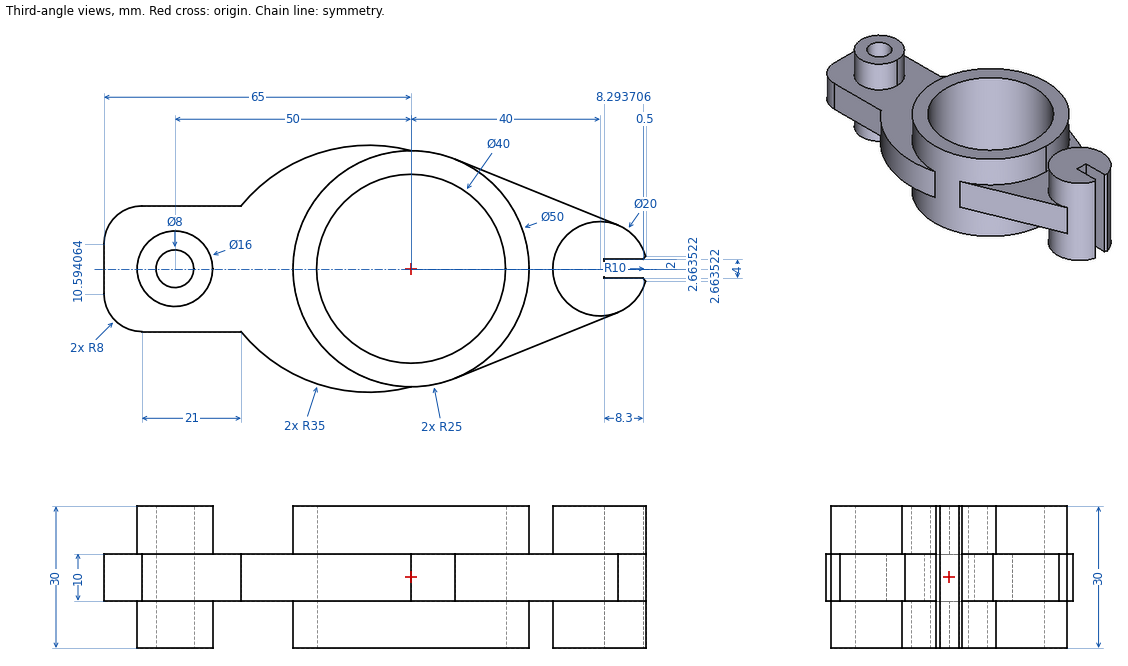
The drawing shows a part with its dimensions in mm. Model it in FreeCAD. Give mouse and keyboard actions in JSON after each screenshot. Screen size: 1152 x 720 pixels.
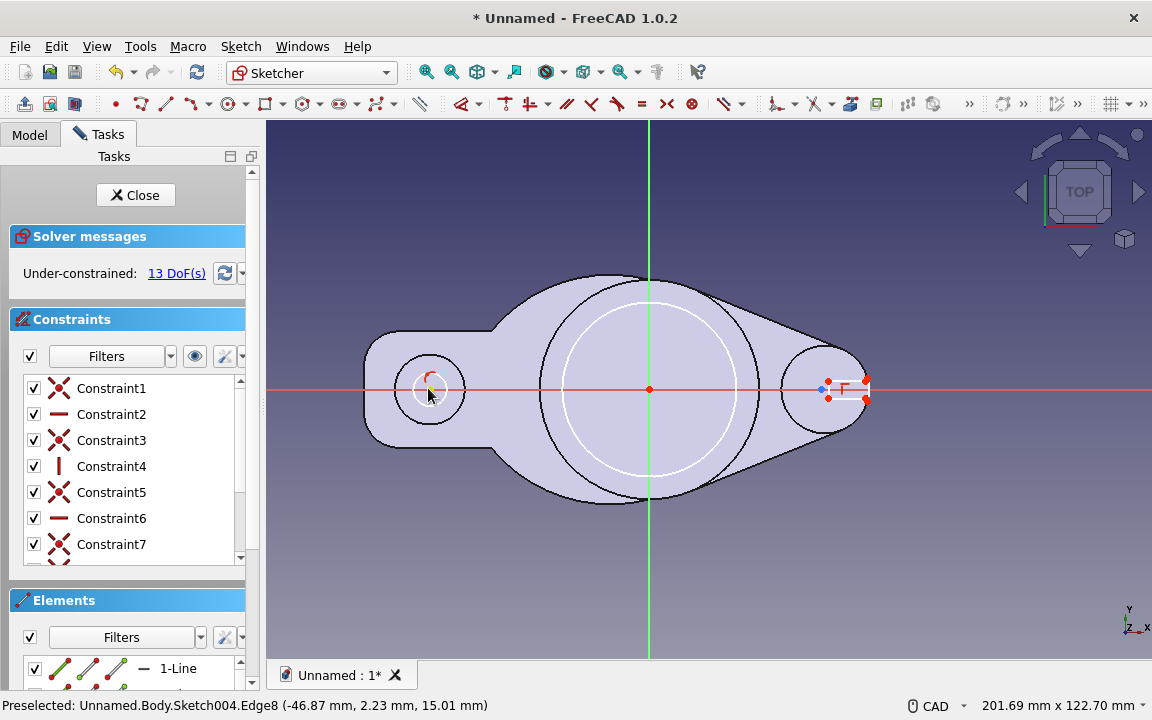
{"action": "left_click", "coordinate": [822, 389]}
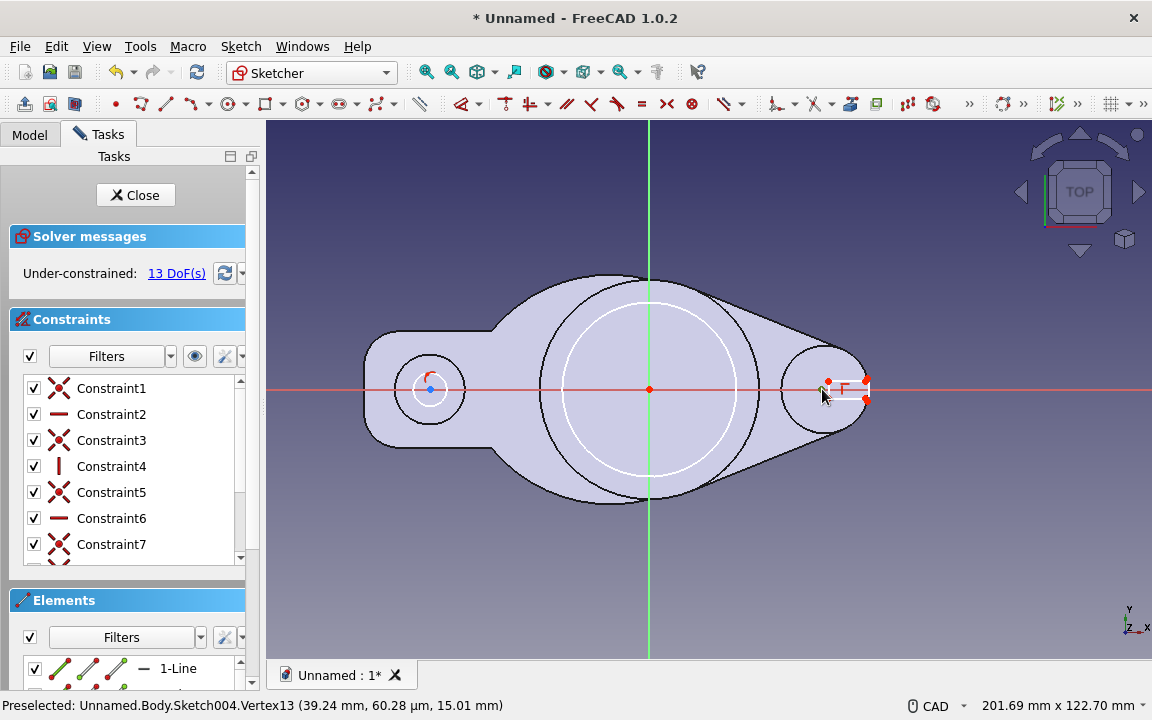
{"action": "left_click", "coordinate": [344, 390]}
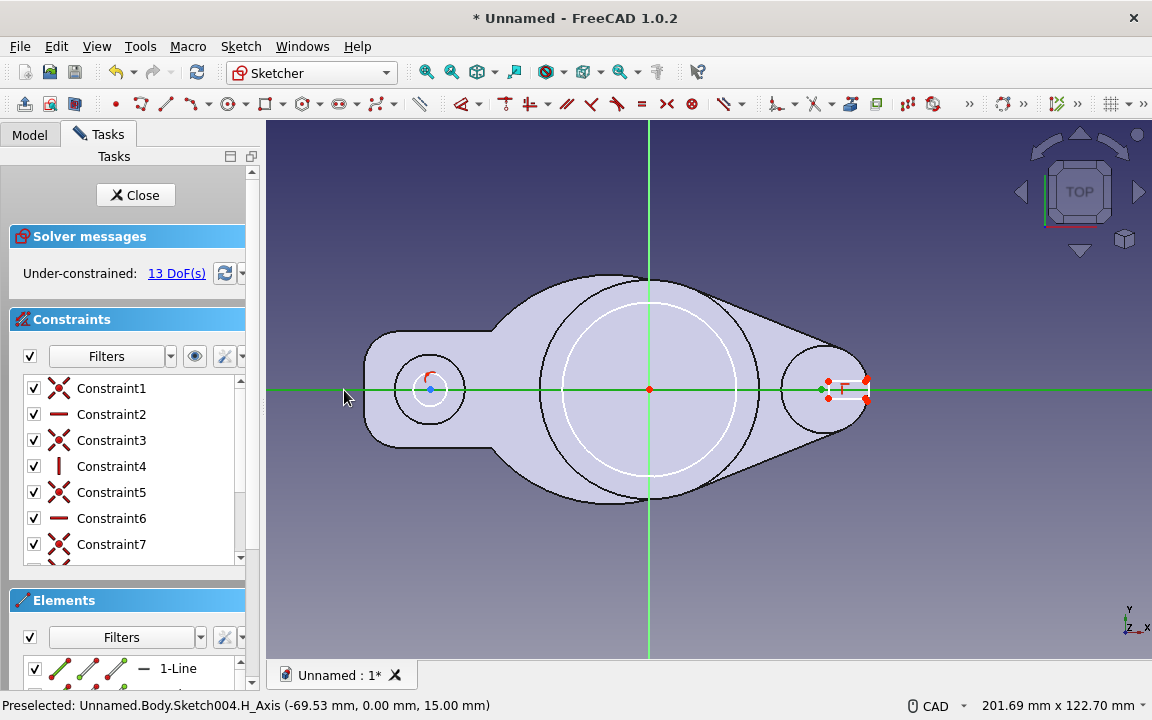
{"action": "left_click", "coordinate": [505, 104]}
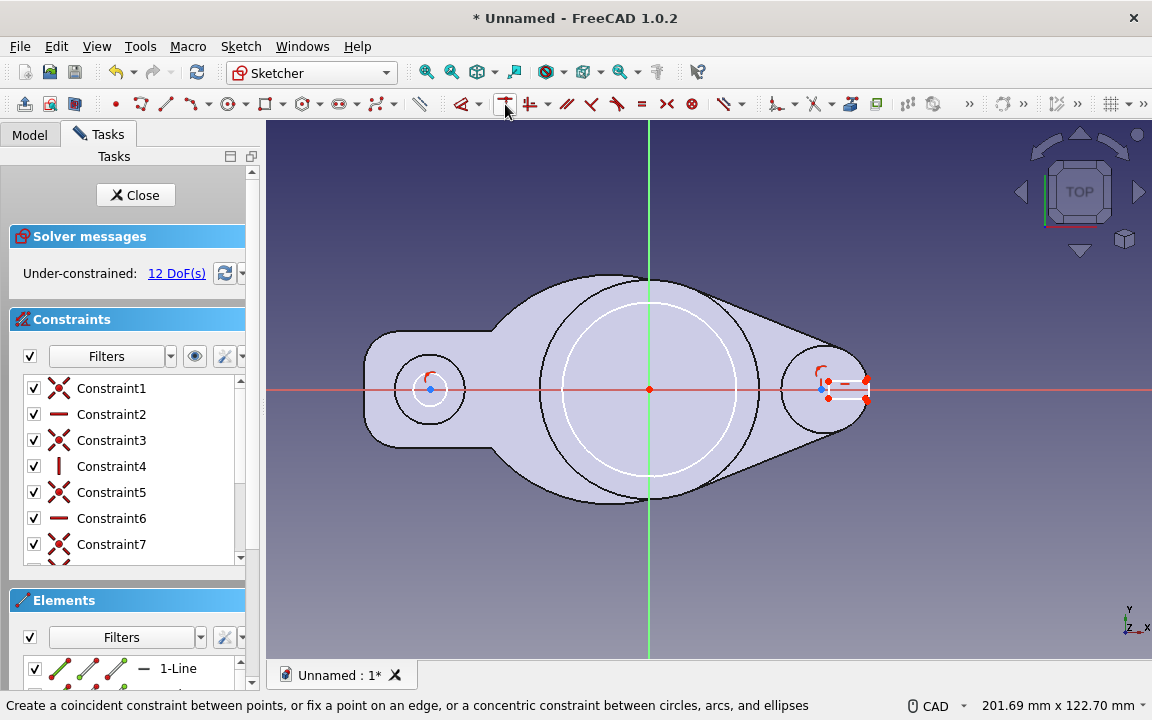
{"action": "left_click", "coordinate": [460, 104]}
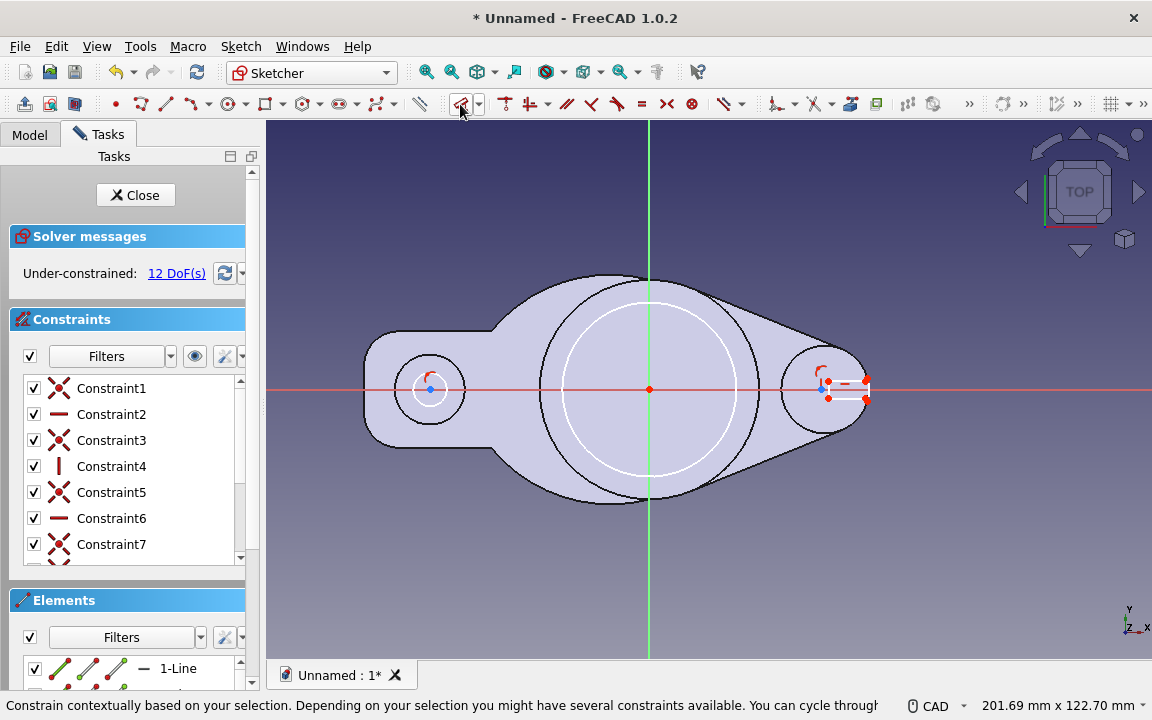
{"action": "scroll", "coordinate": [869, 390], "scroll_direction": "up", "scroll_amount": 2}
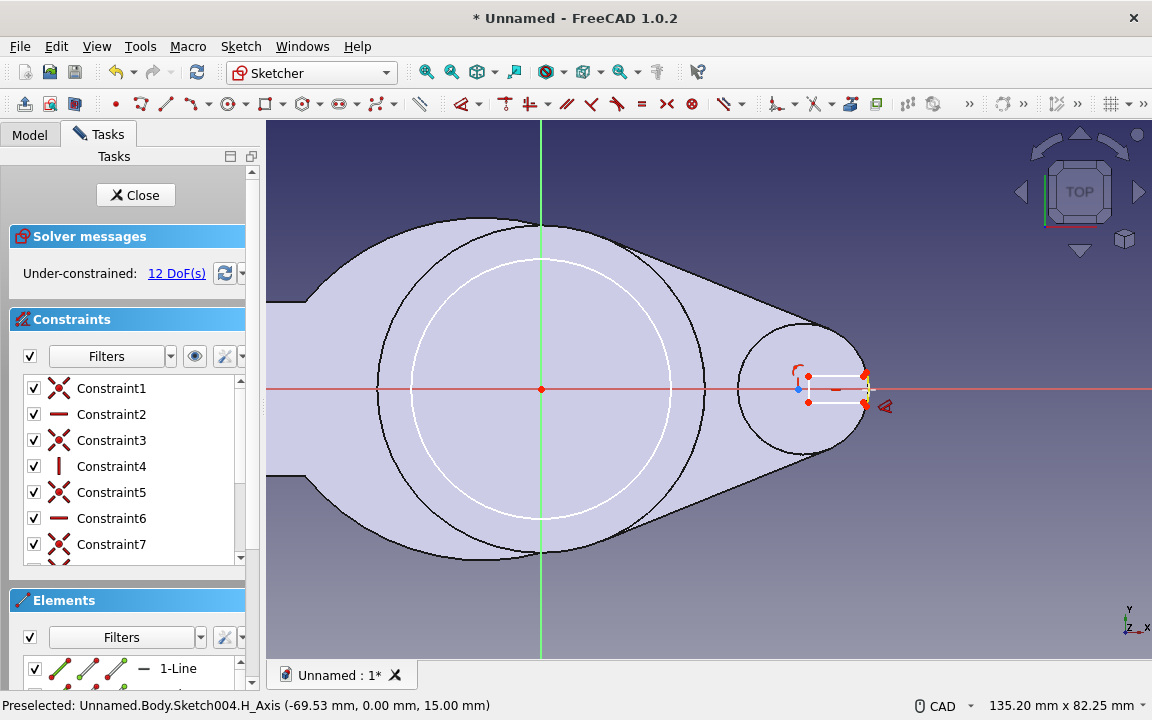
{"action": "left_click", "coordinate": [869, 390]}
{"action": "left_click", "coordinate": [888, 440]}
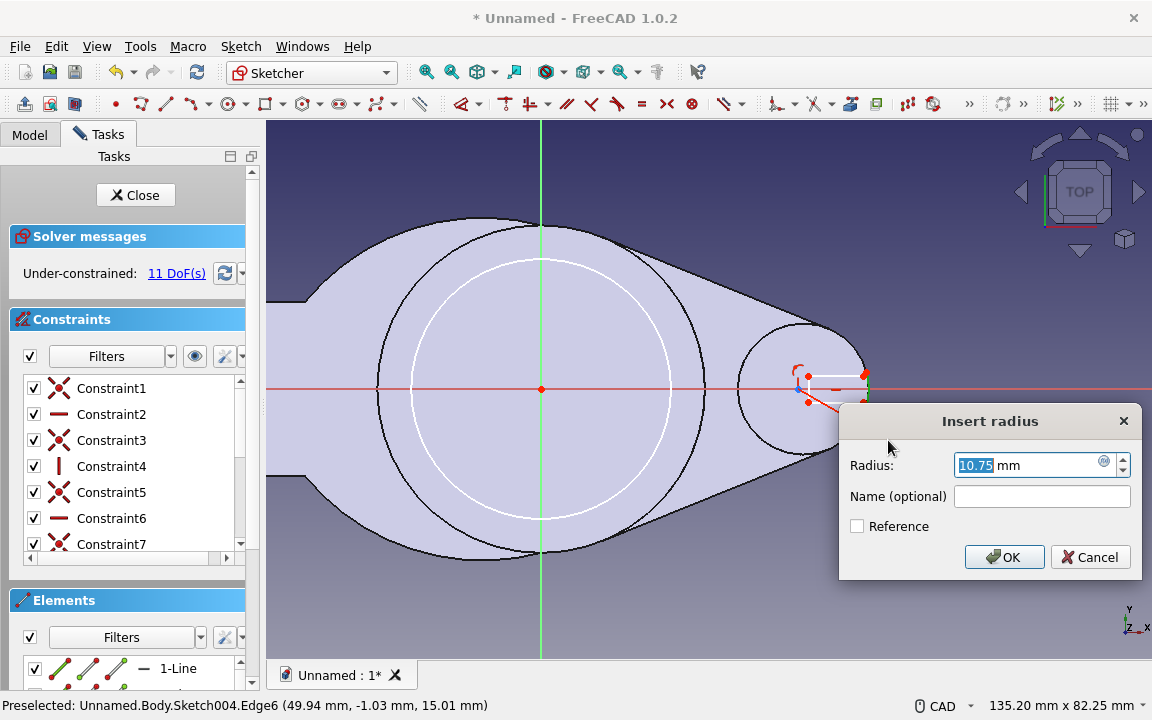
{"action": "type", "text": "10"}
{"action": "key", "text": "Return"}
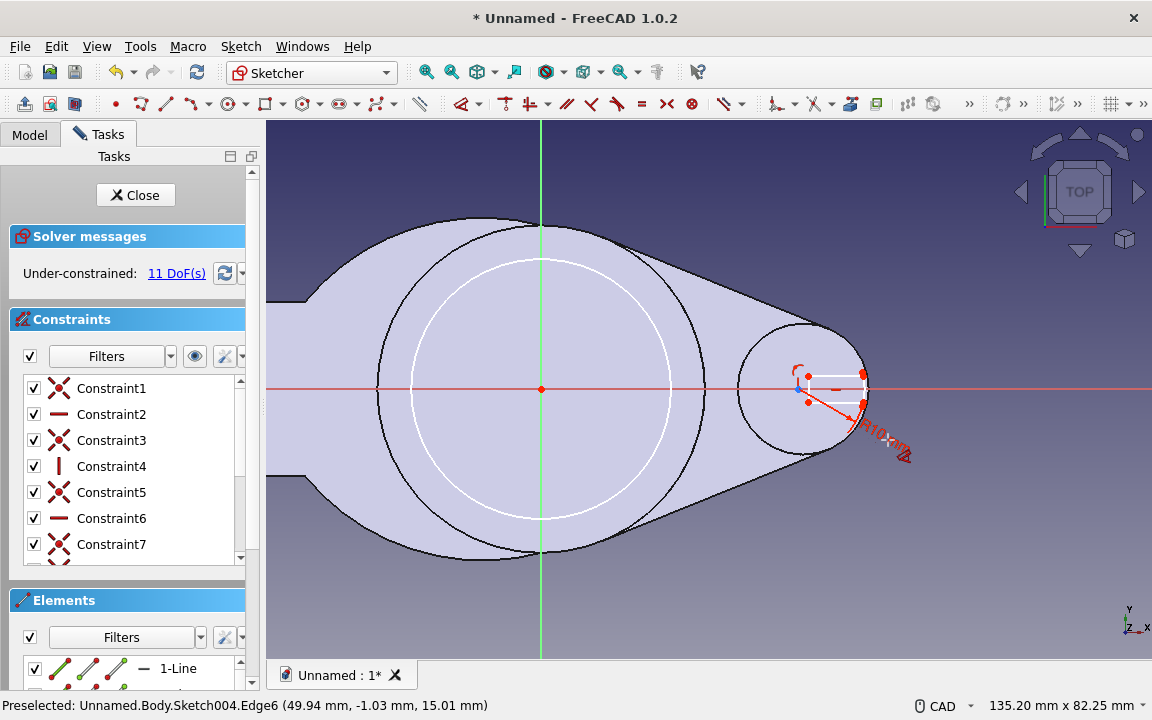
{"action": "left_click", "coordinate": [633, 297]}
{"action": "left_click", "coordinate": [656, 274]}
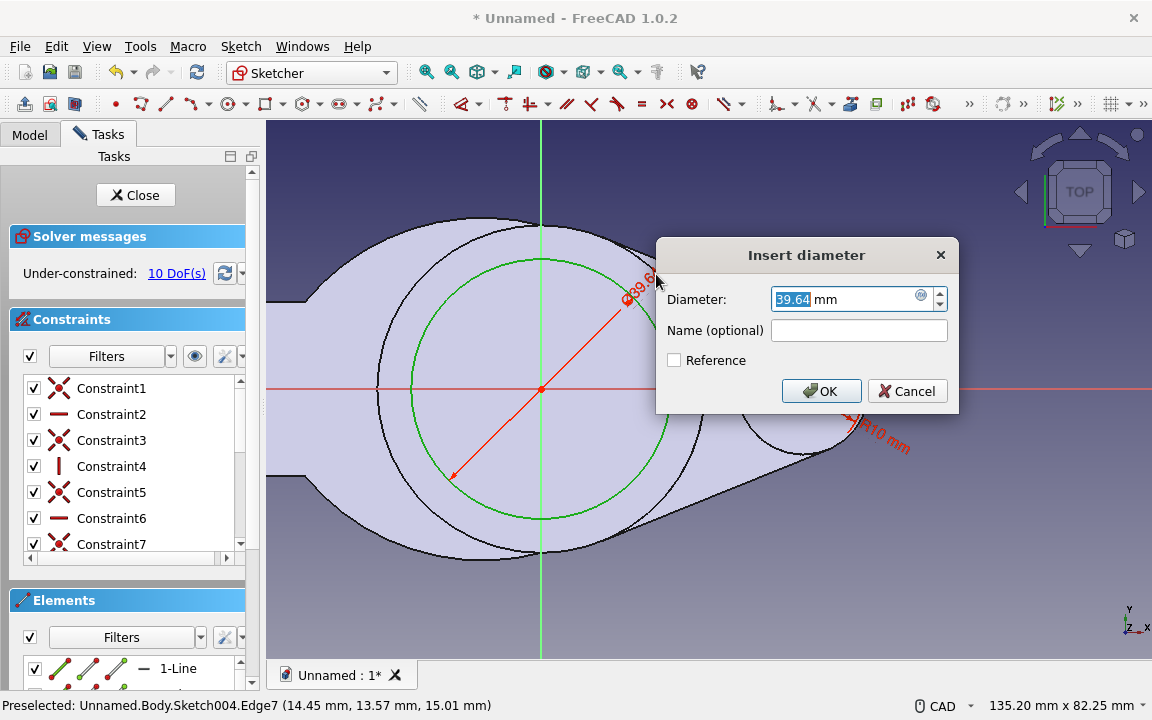
{"action": "type", "text": "40"}
{"action": "key", "text": "Return"}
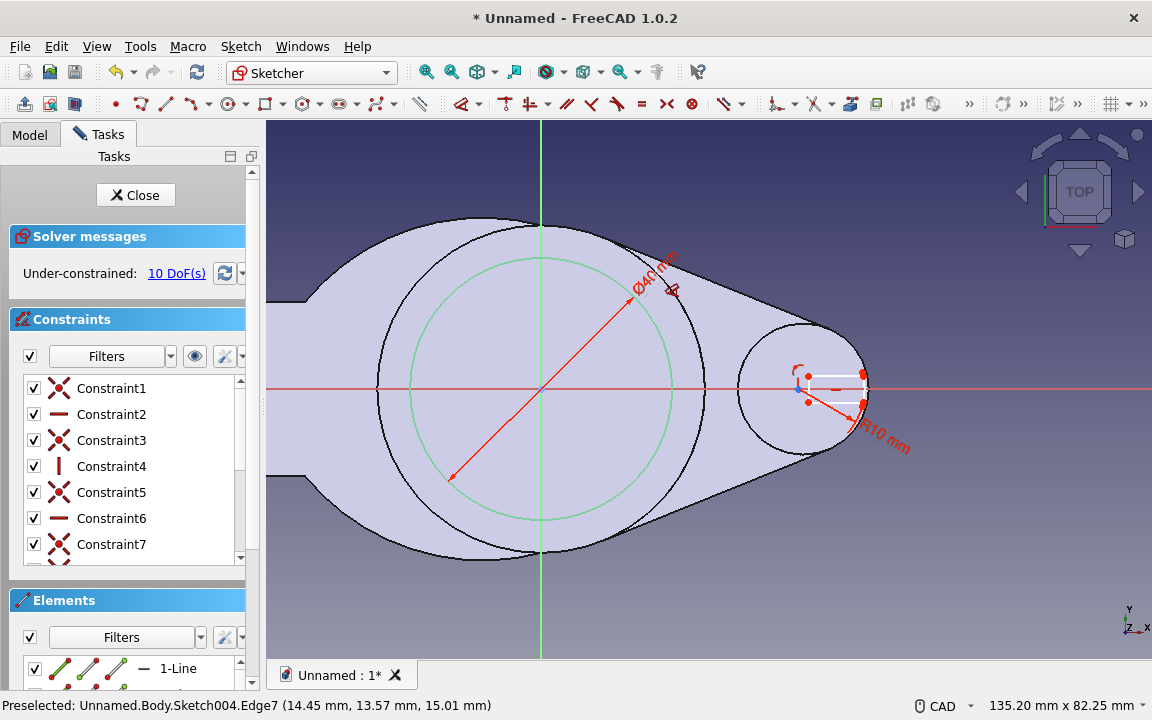
{"action": "scroll", "coordinate": [869, 390], "scroll_direction": "down", "scroll_amount": 2}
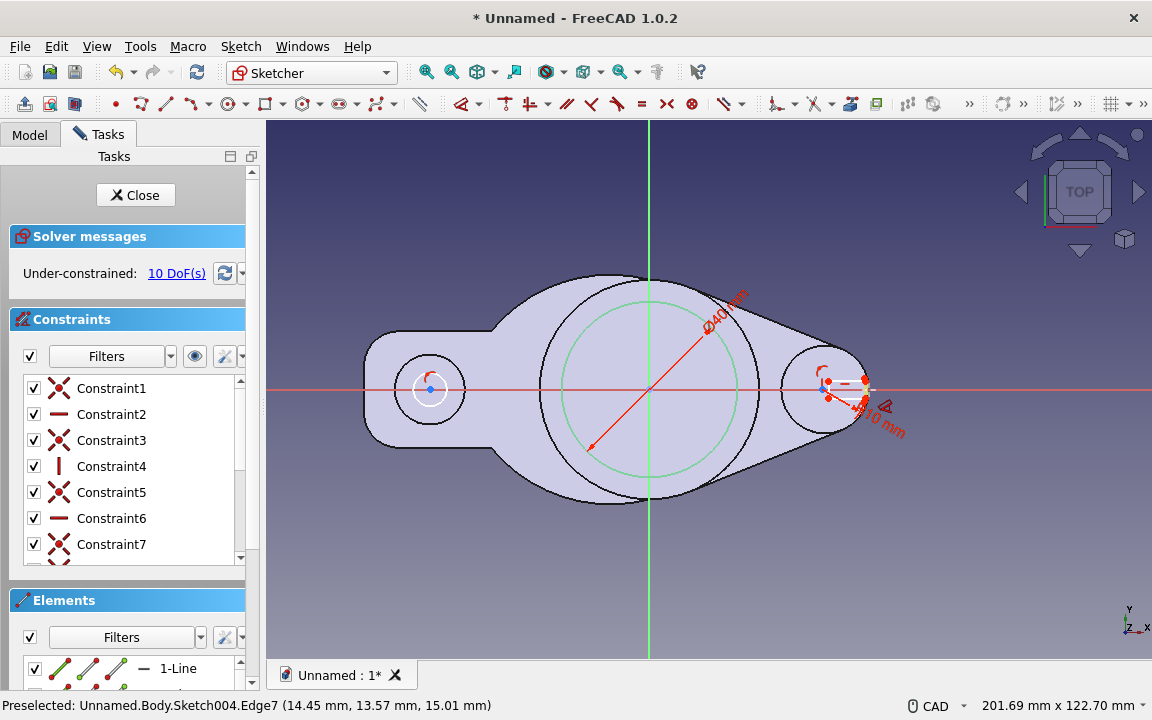
{"action": "left_click", "coordinate": [442, 378]}
{"action": "left_click", "coordinate": [465, 356]}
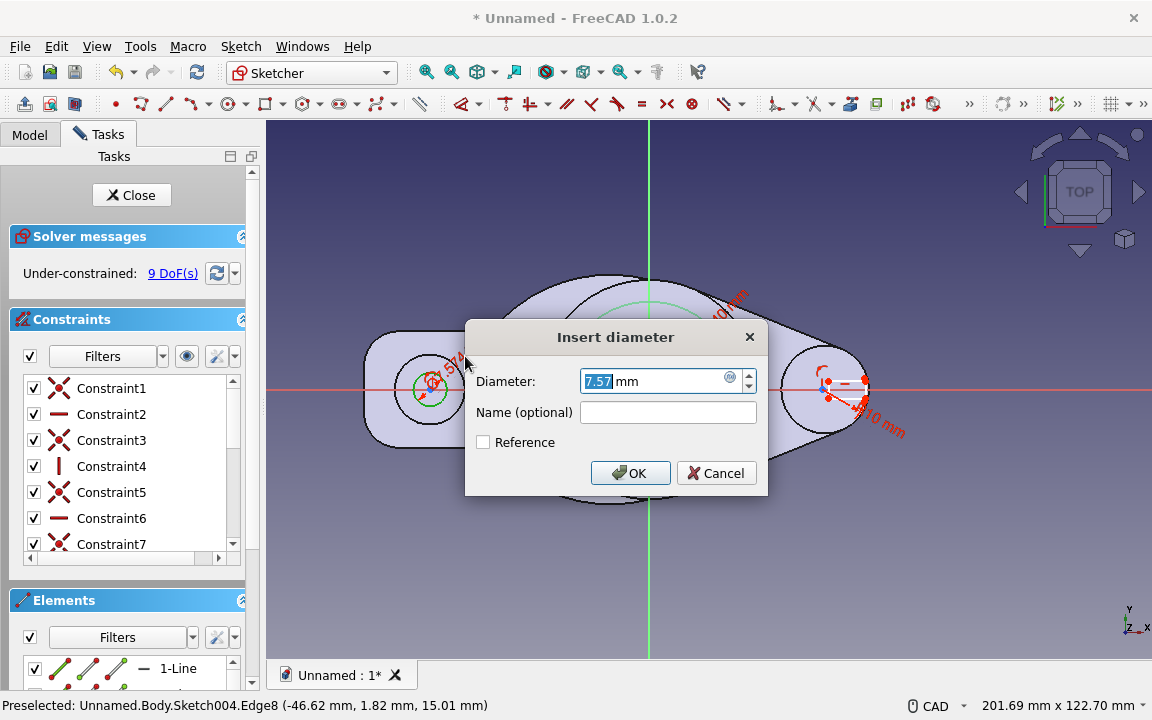
{"action": "type", "text": "8"}
{"action": "key", "text": "Return"}